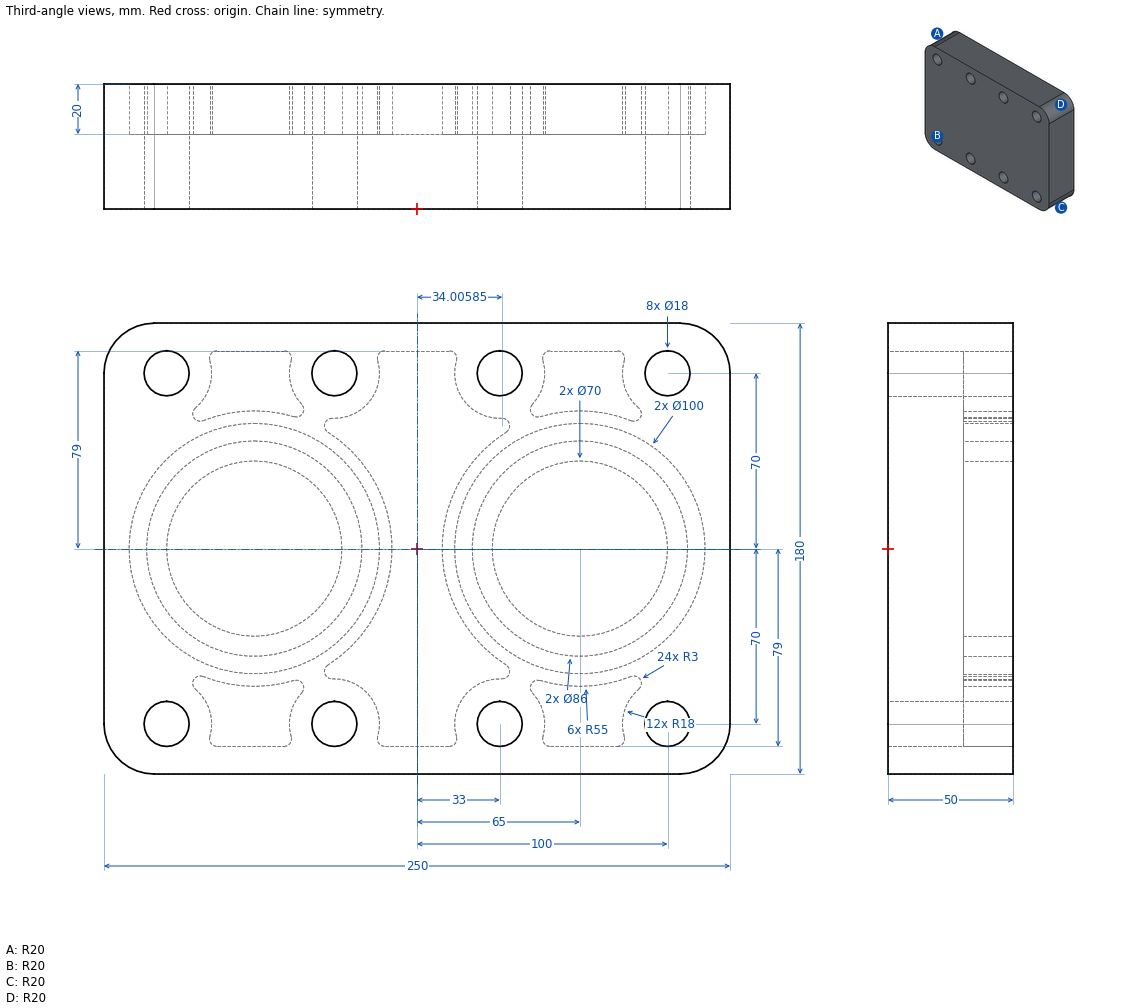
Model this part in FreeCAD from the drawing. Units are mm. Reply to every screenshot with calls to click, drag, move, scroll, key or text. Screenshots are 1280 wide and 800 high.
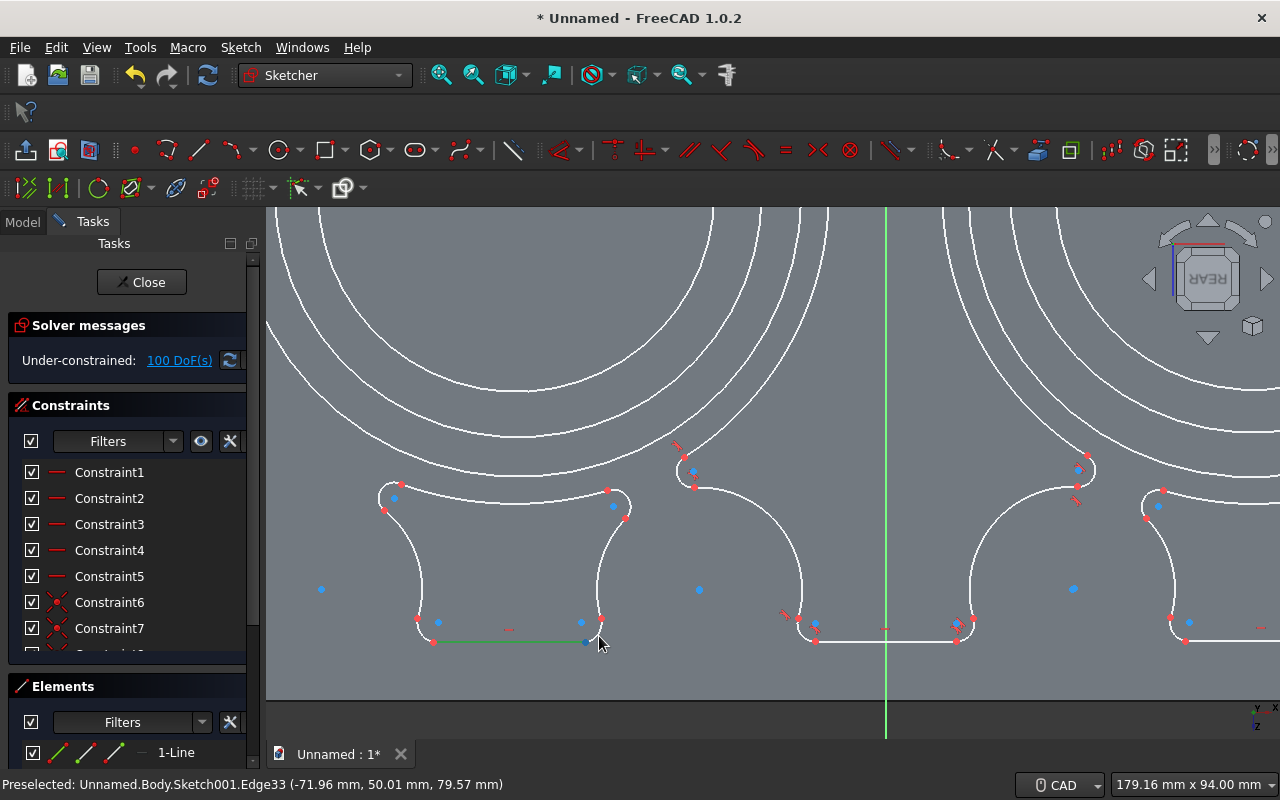
click(598, 634)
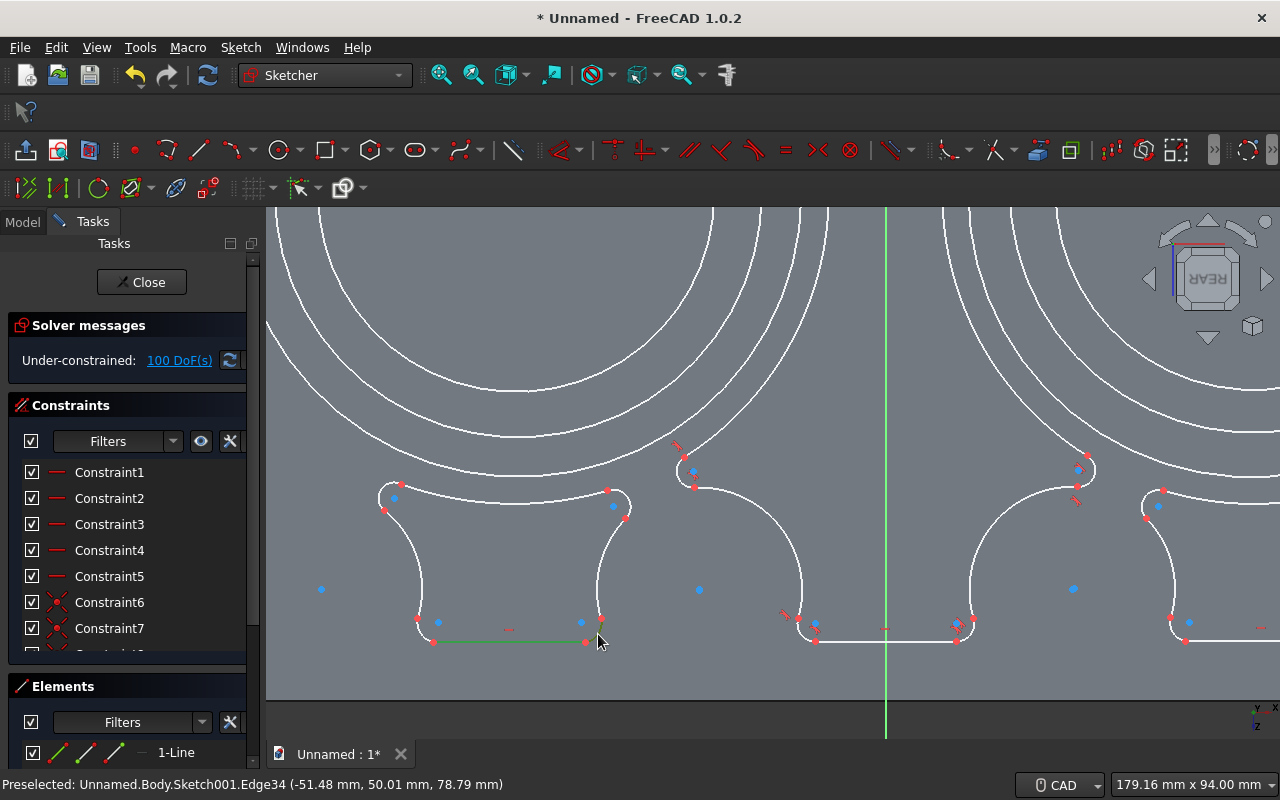
click(754, 150)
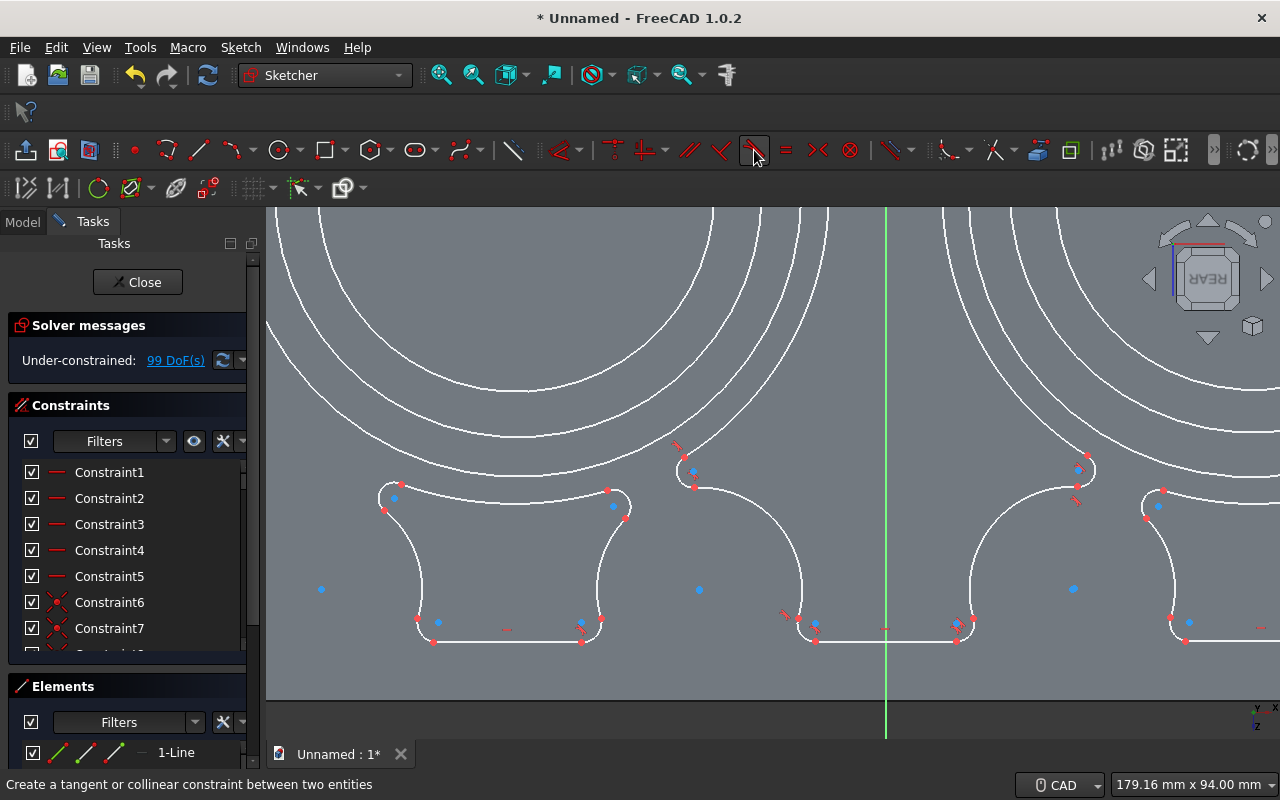
click(478, 642)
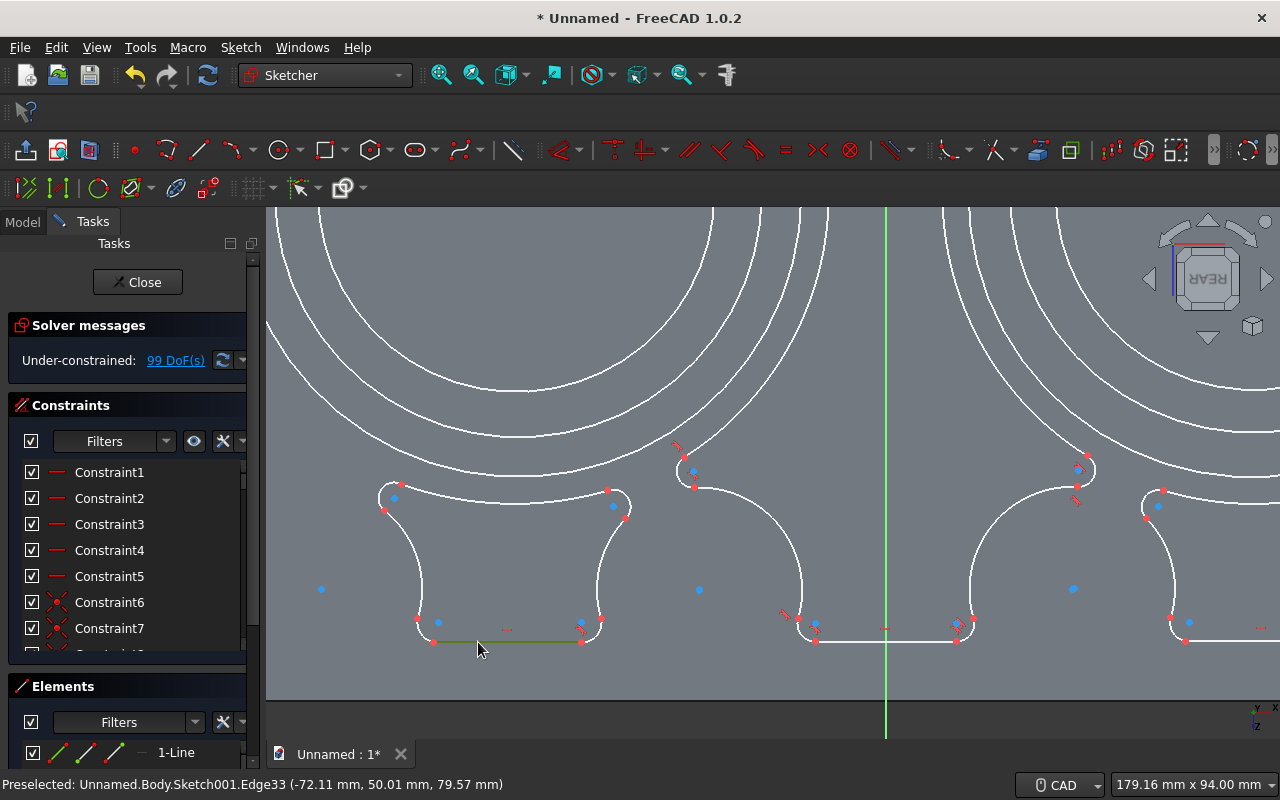
scroll(418, 628, up, 2)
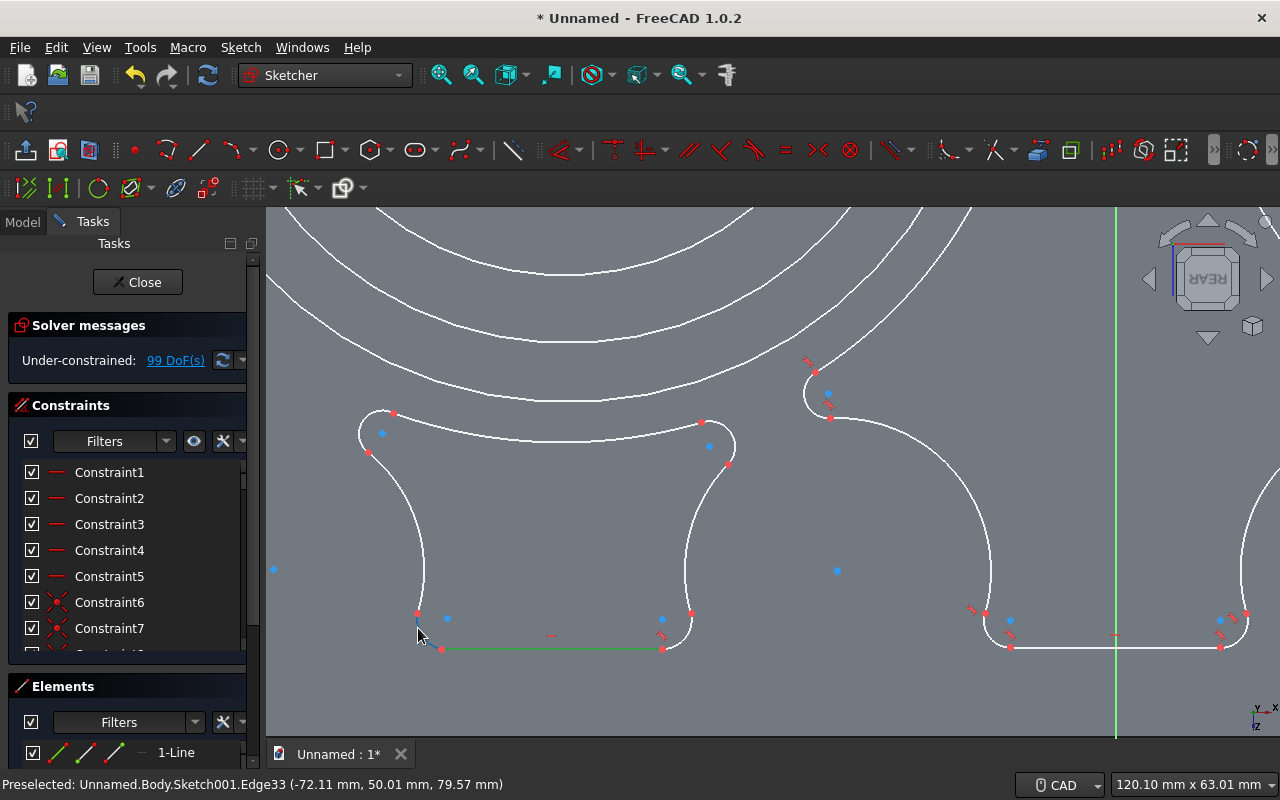
click(418, 628)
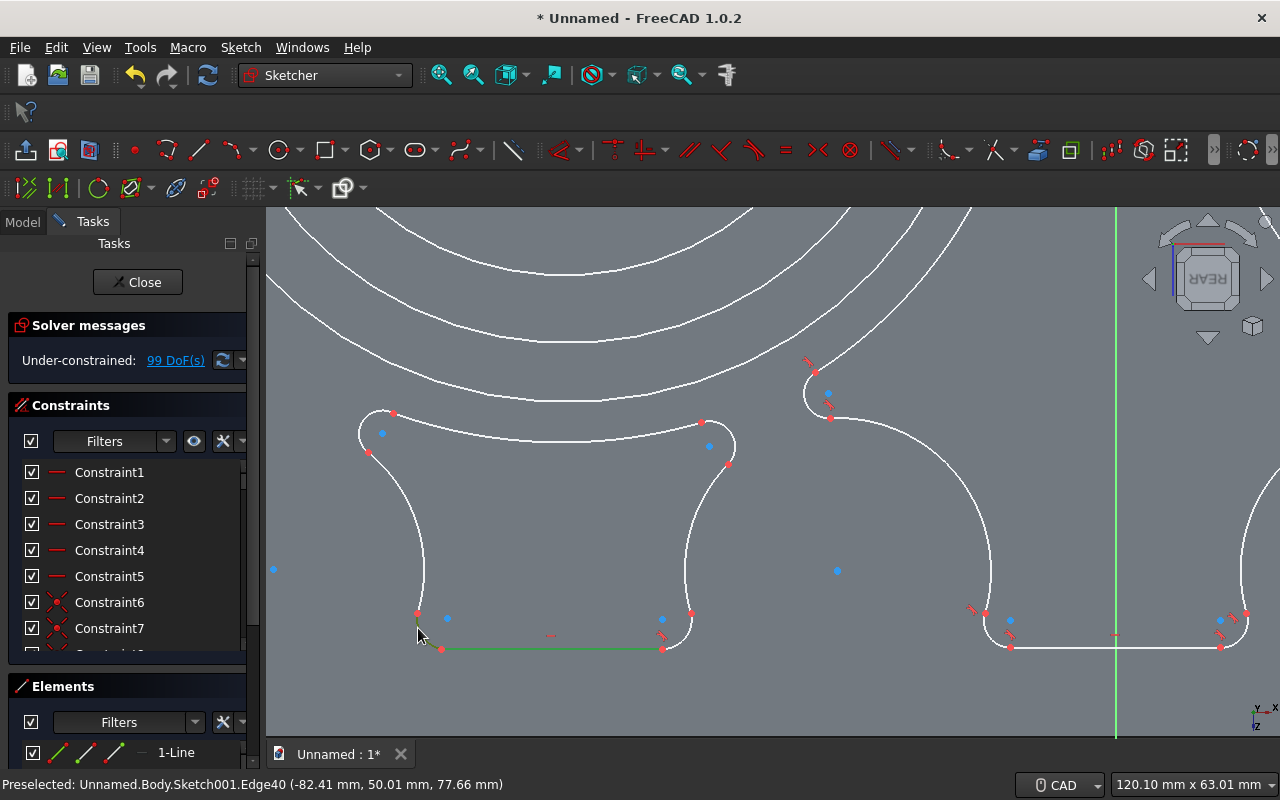
click(754, 150)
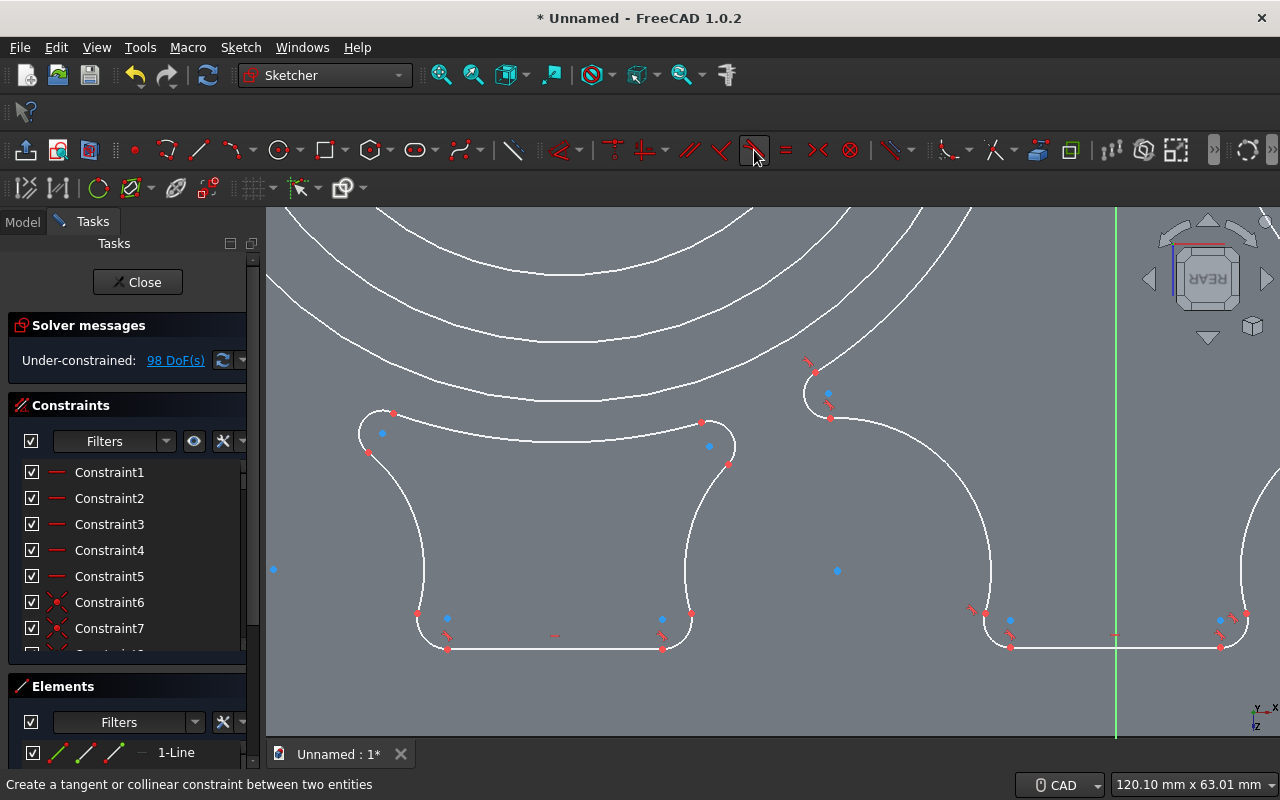
click(677, 645)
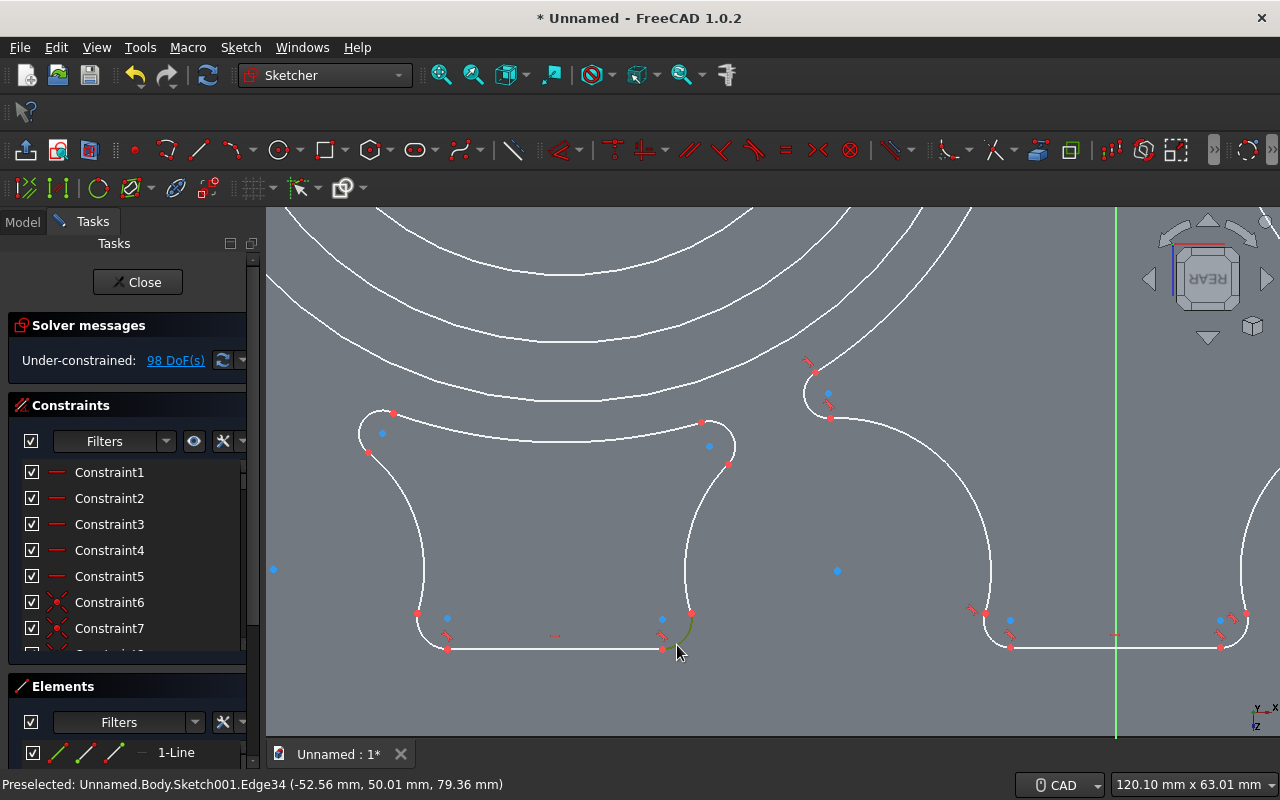
scroll(570, 635, down, 7)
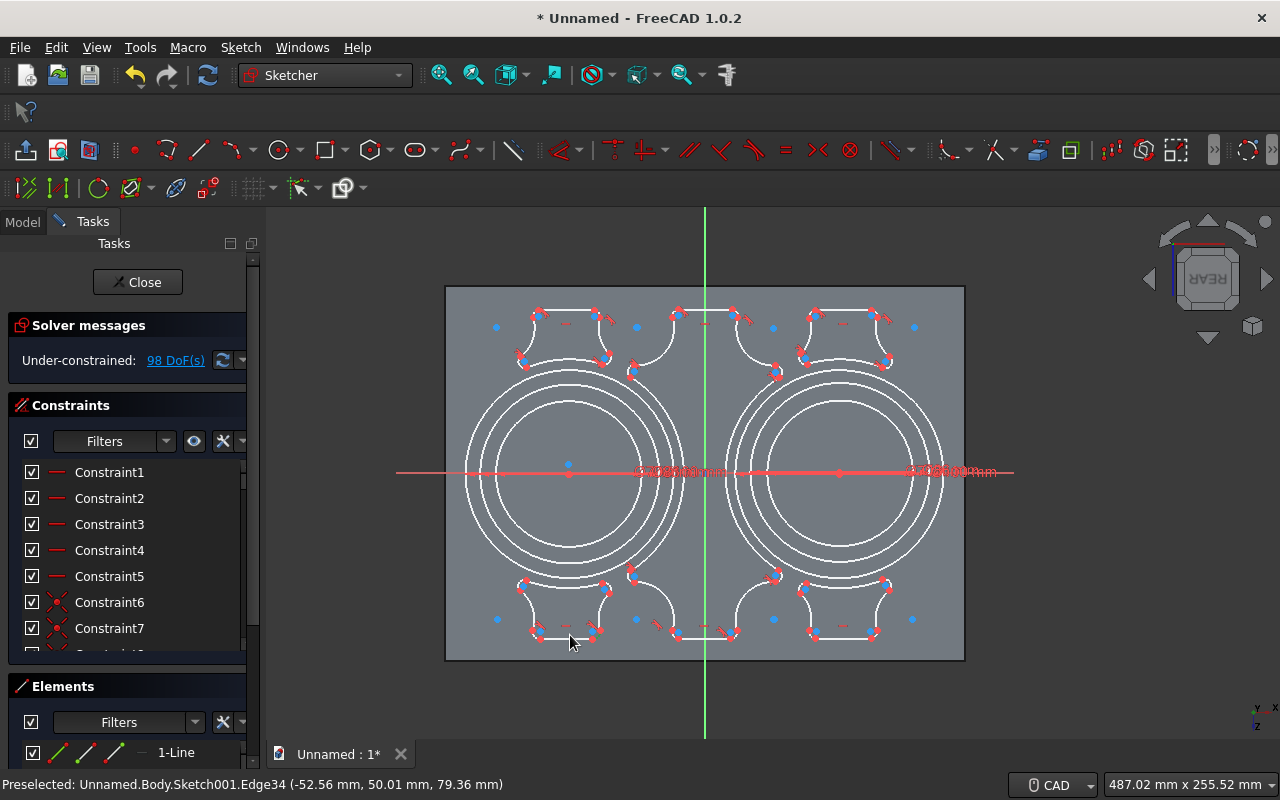
click(602, 603)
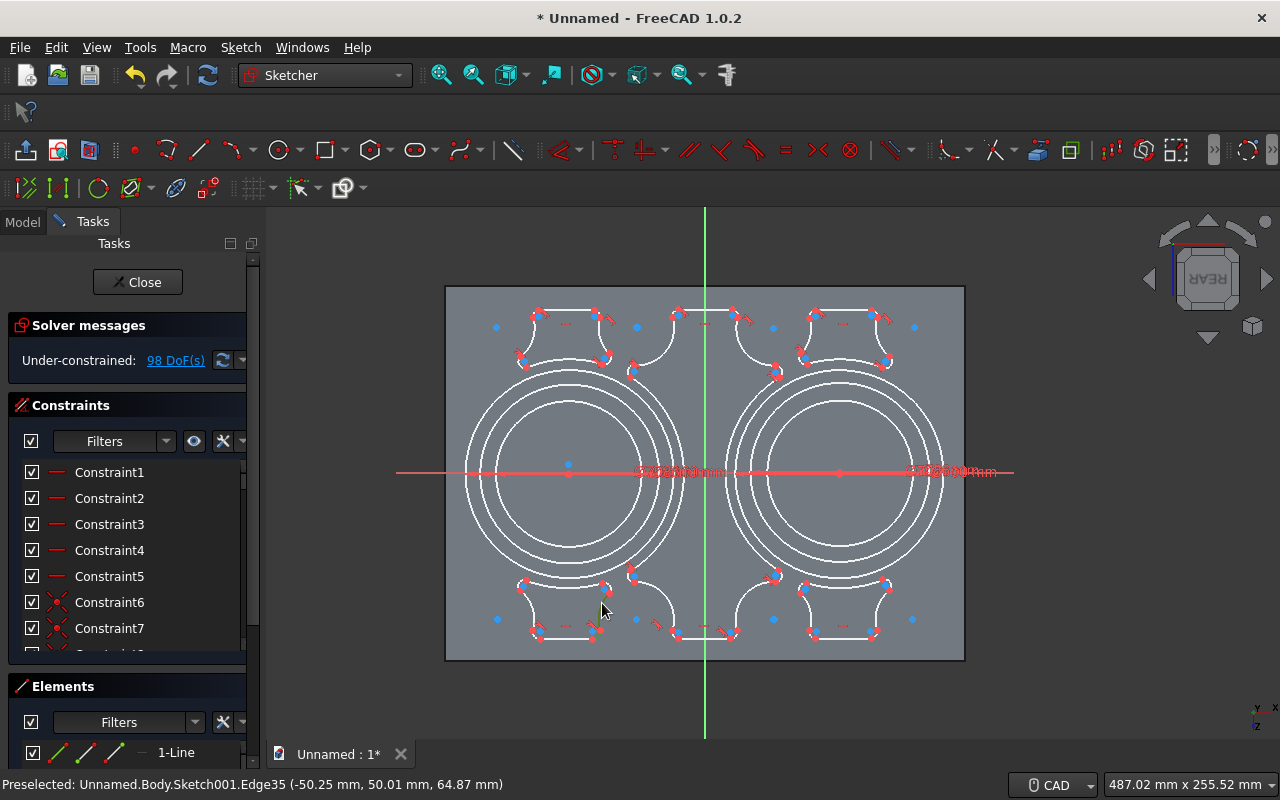
click(754, 150)